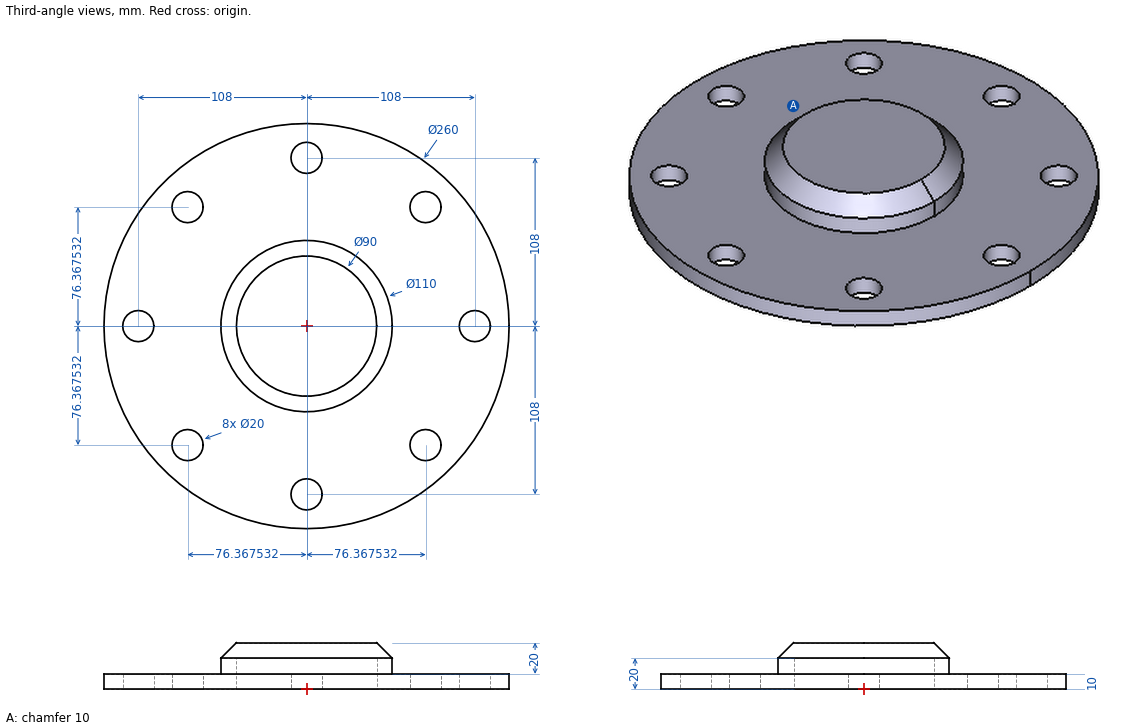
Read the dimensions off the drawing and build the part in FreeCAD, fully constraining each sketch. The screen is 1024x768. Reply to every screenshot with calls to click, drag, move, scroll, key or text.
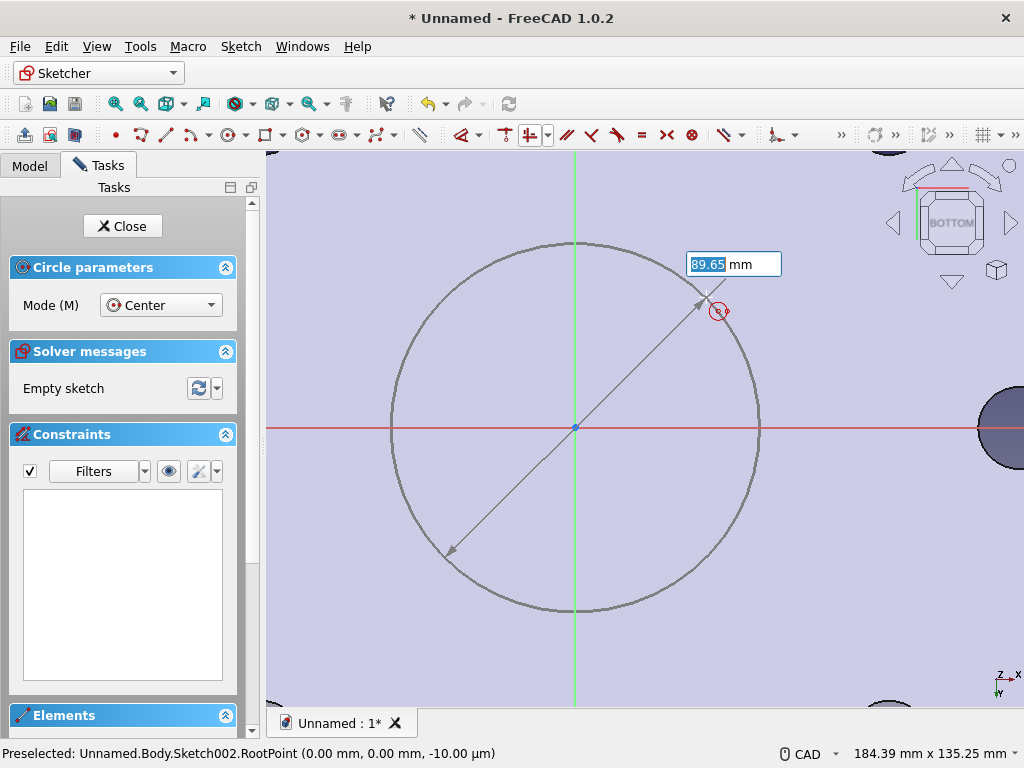
text(90)
key(Return)
key(Escape)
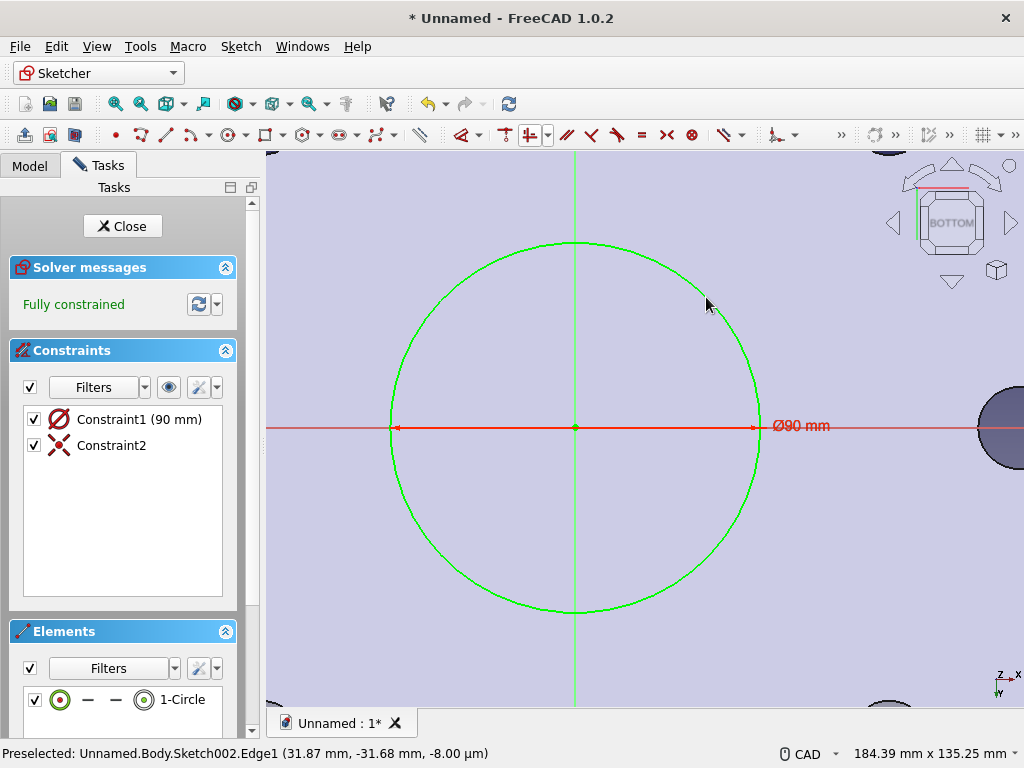
click(123, 226)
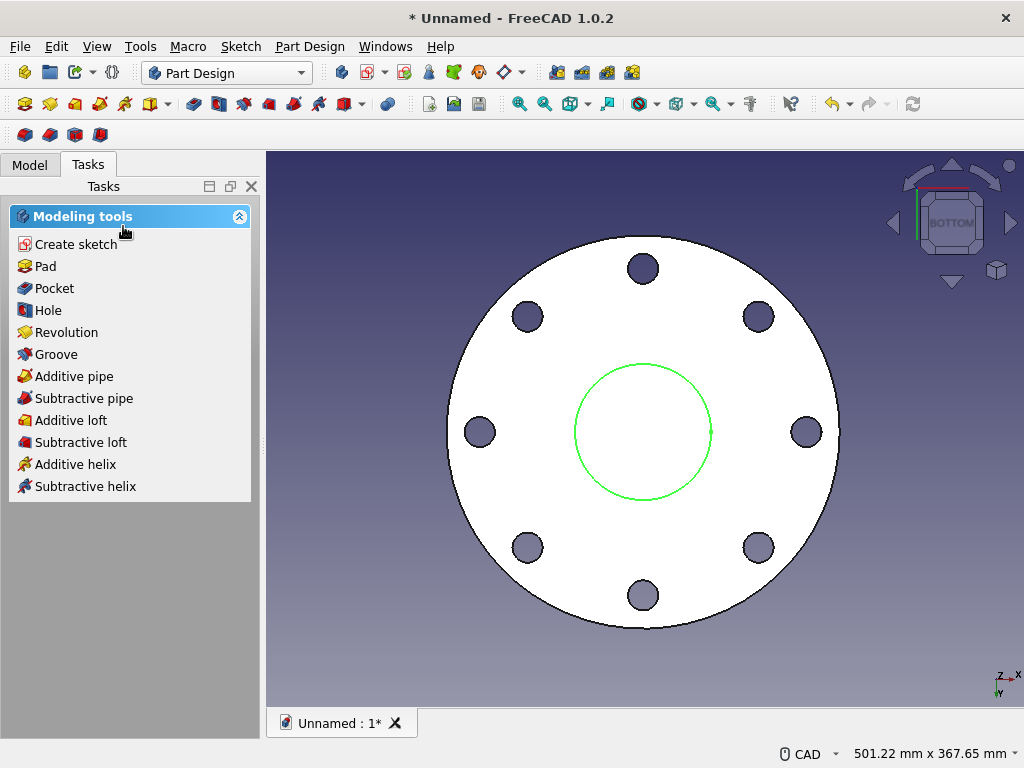
click(194, 104)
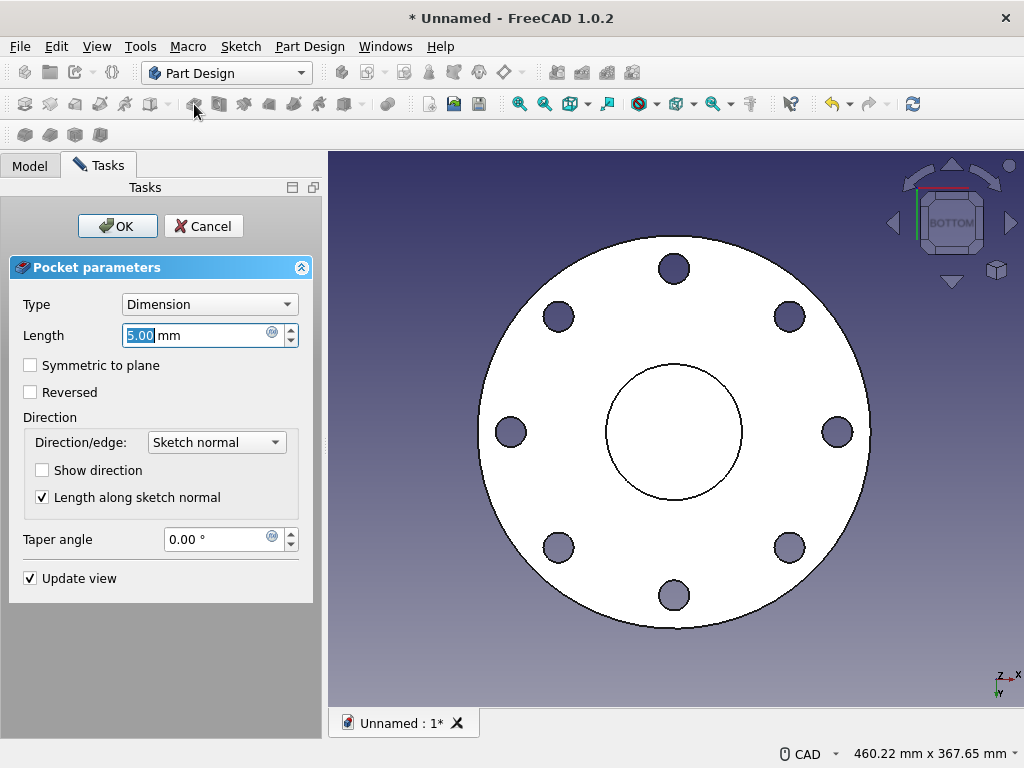
text(20)
key(Tab)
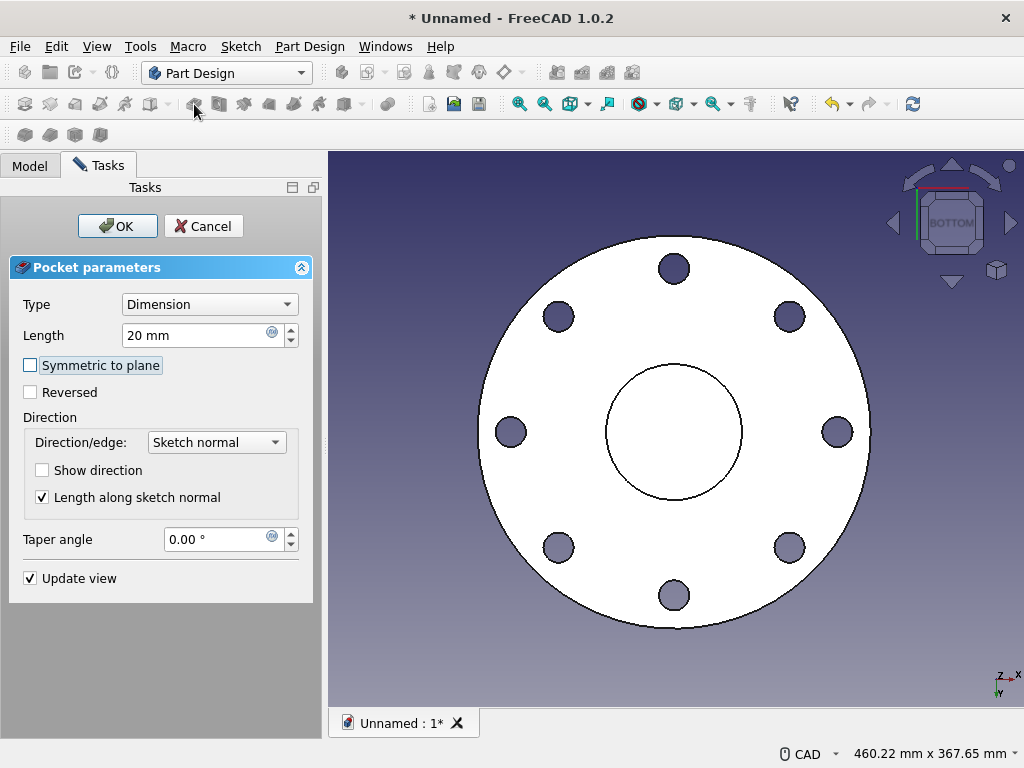
click(118, 226)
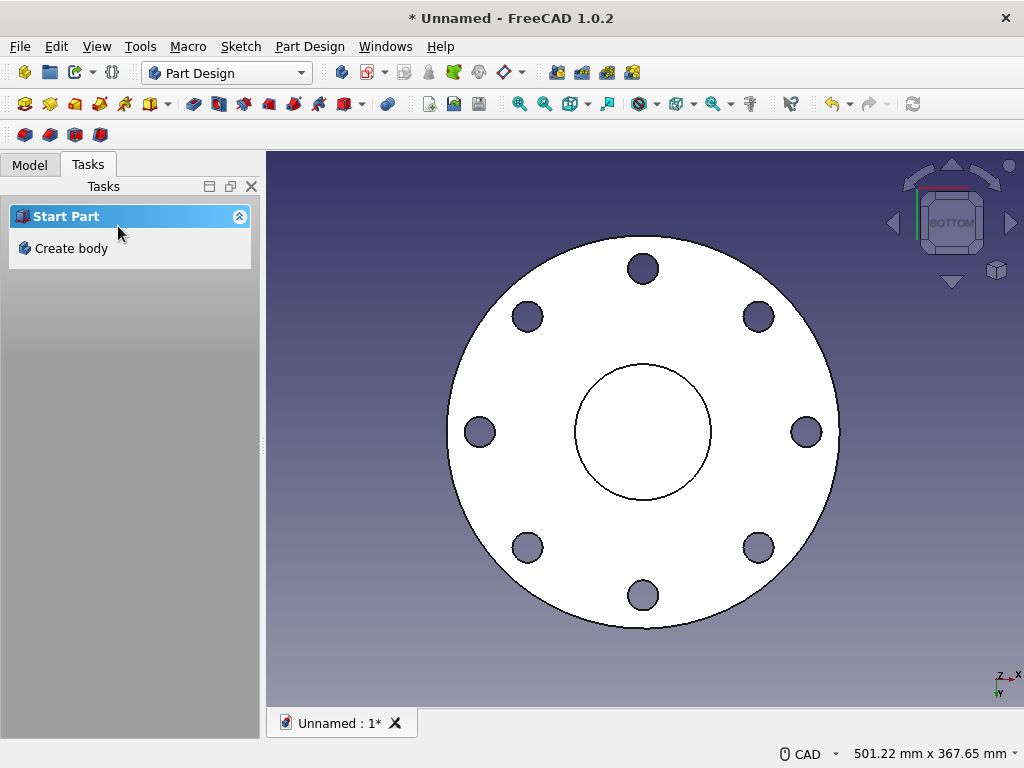
key(0)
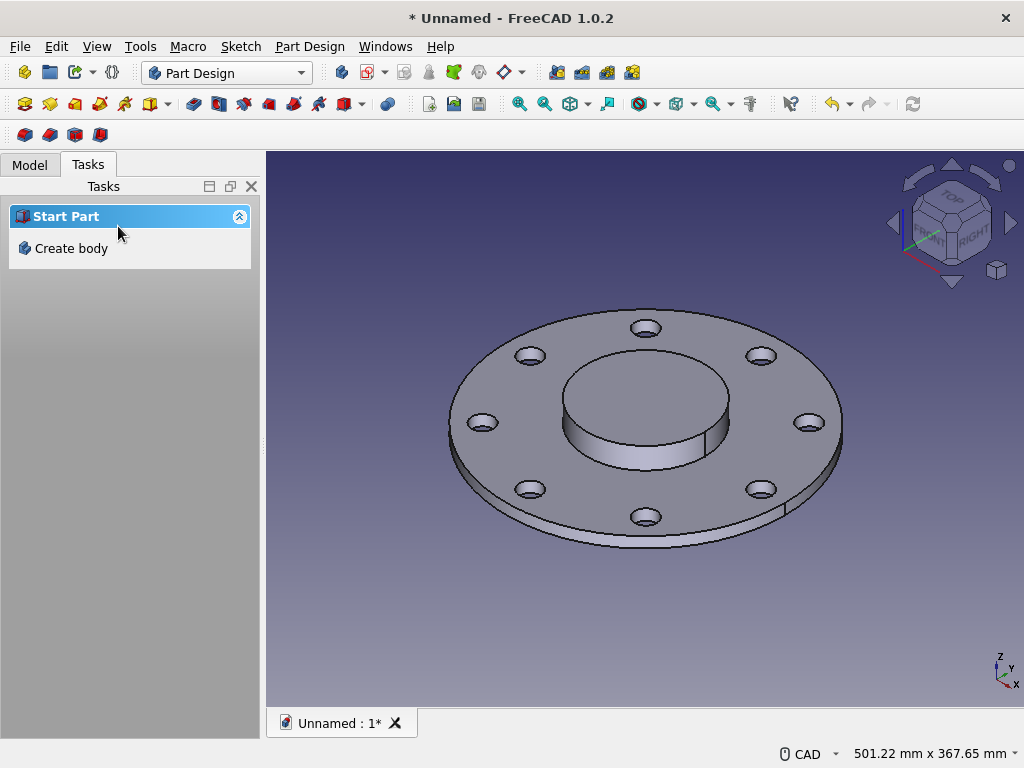
click(572, 419)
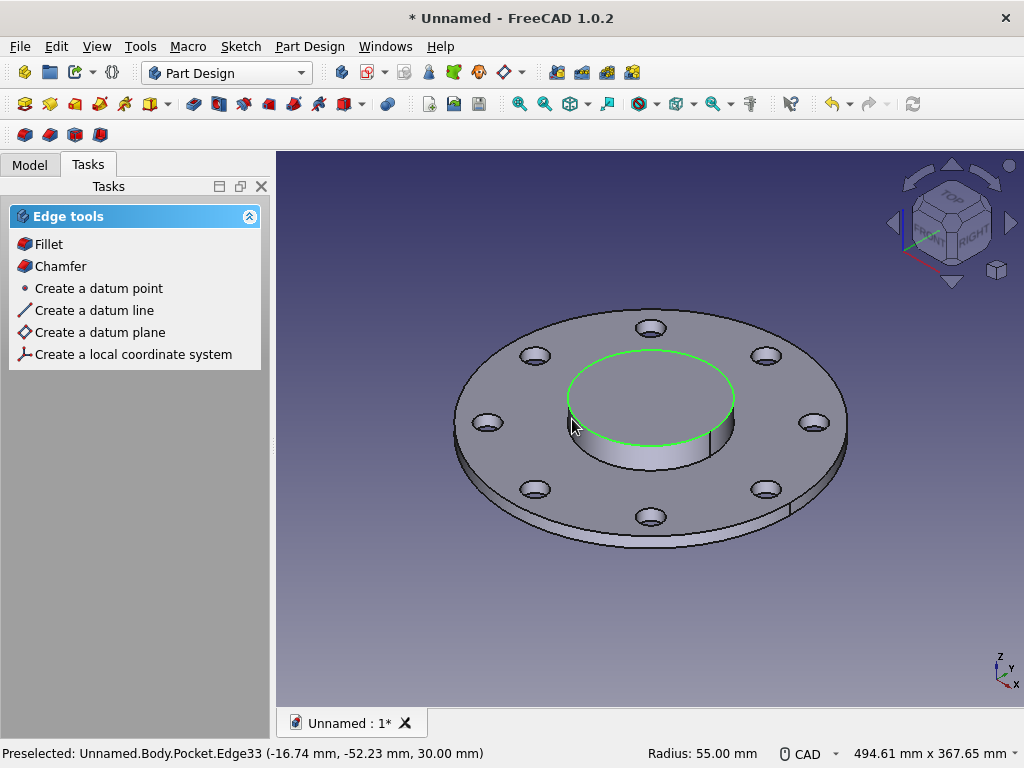
click(50, 136)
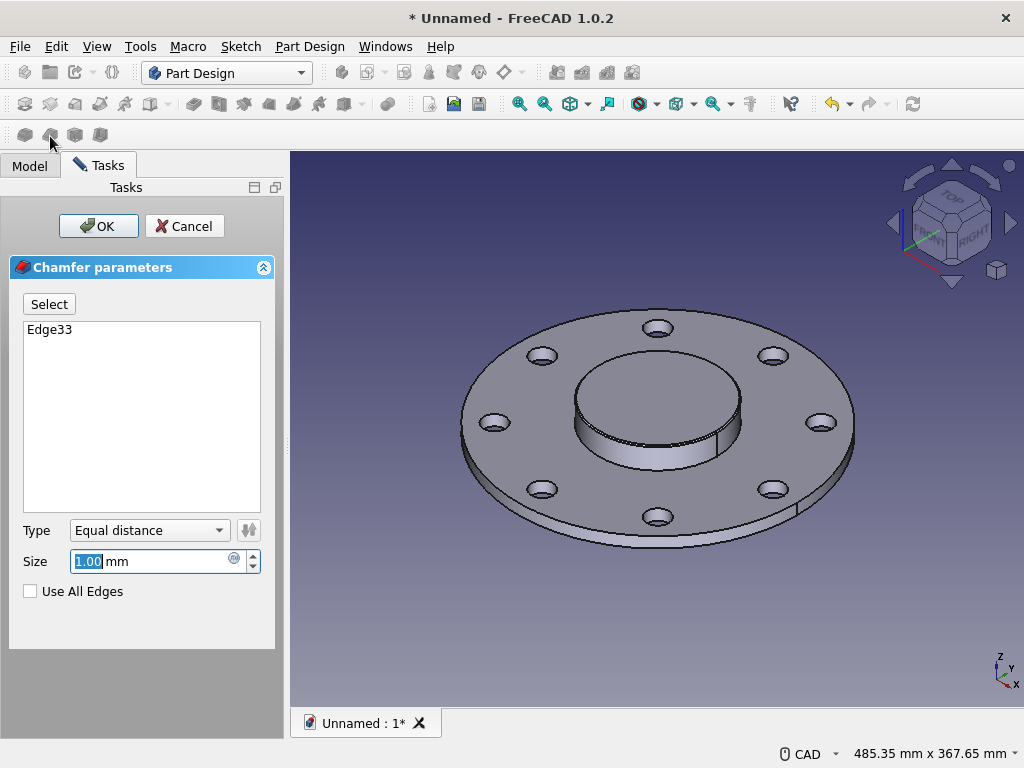
text(10)
key(Tab)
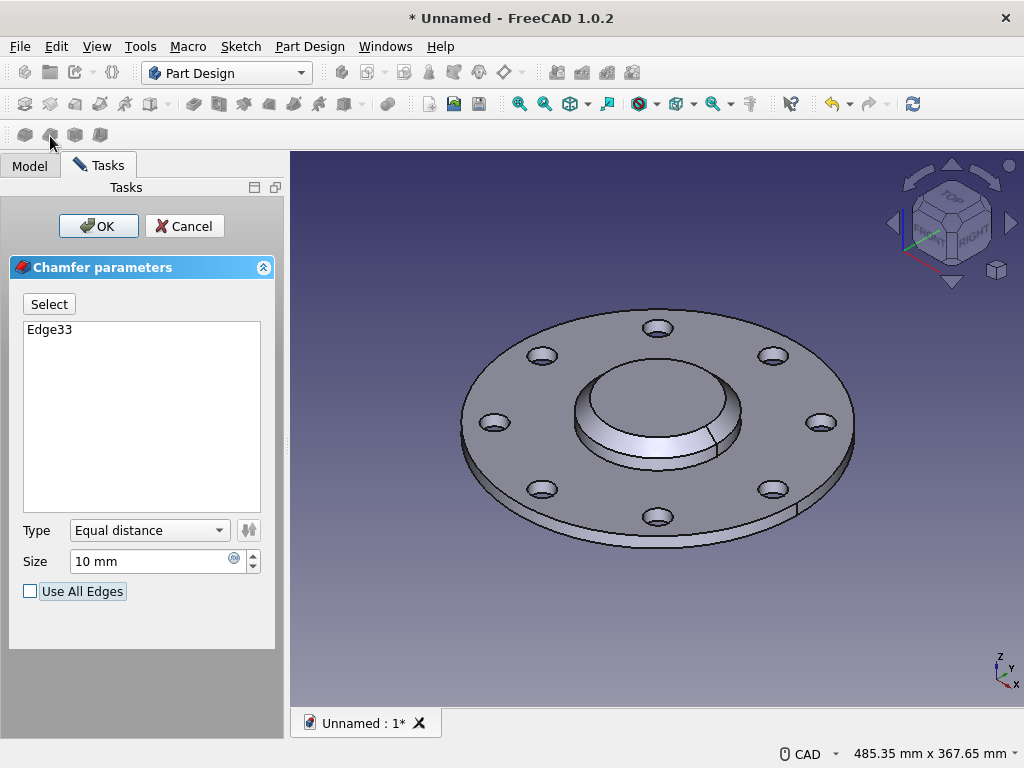
click(99, 226)